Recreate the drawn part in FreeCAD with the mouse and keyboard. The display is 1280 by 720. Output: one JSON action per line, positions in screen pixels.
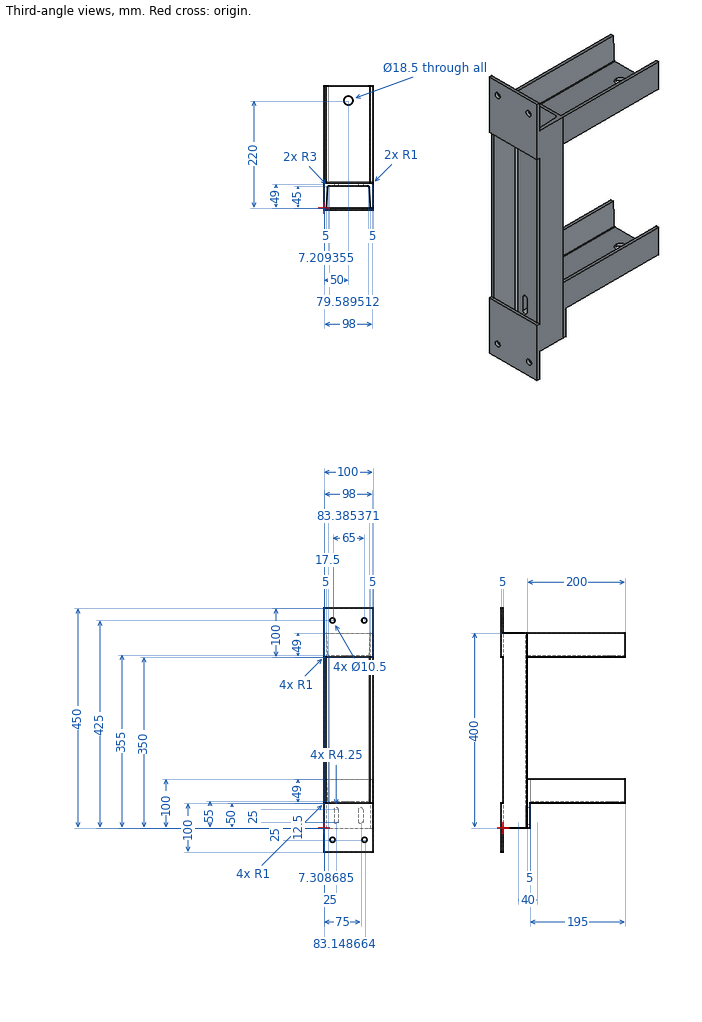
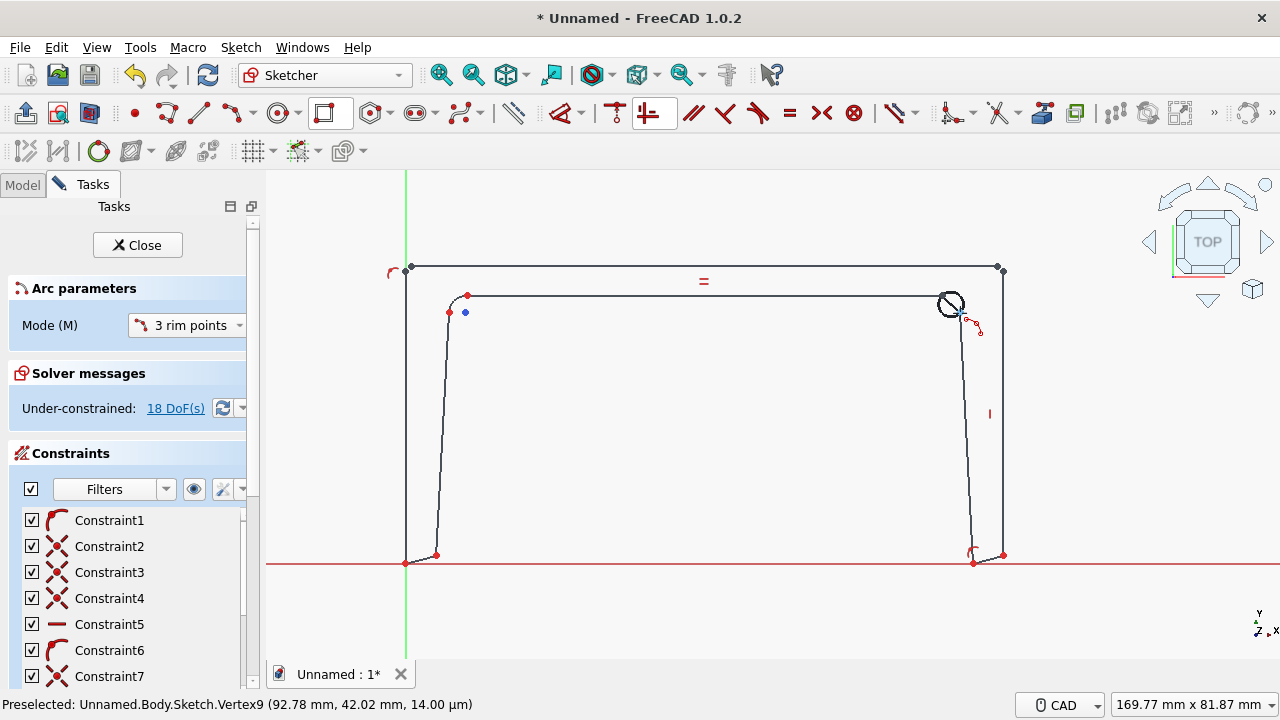
{"action": "scroll", "coordinate": [955, 300], "scroll_direction": "up", "scroll_amount": 6}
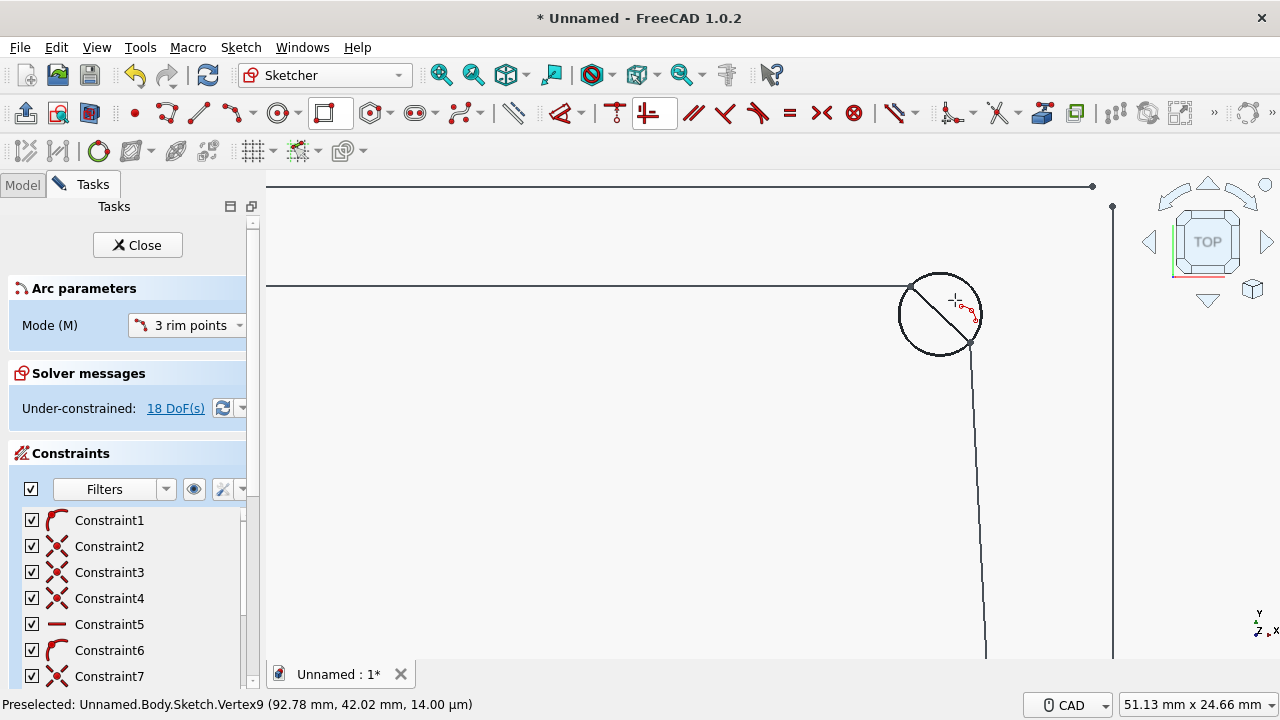
{"action": "left_click", "coordinate": [952, 300]}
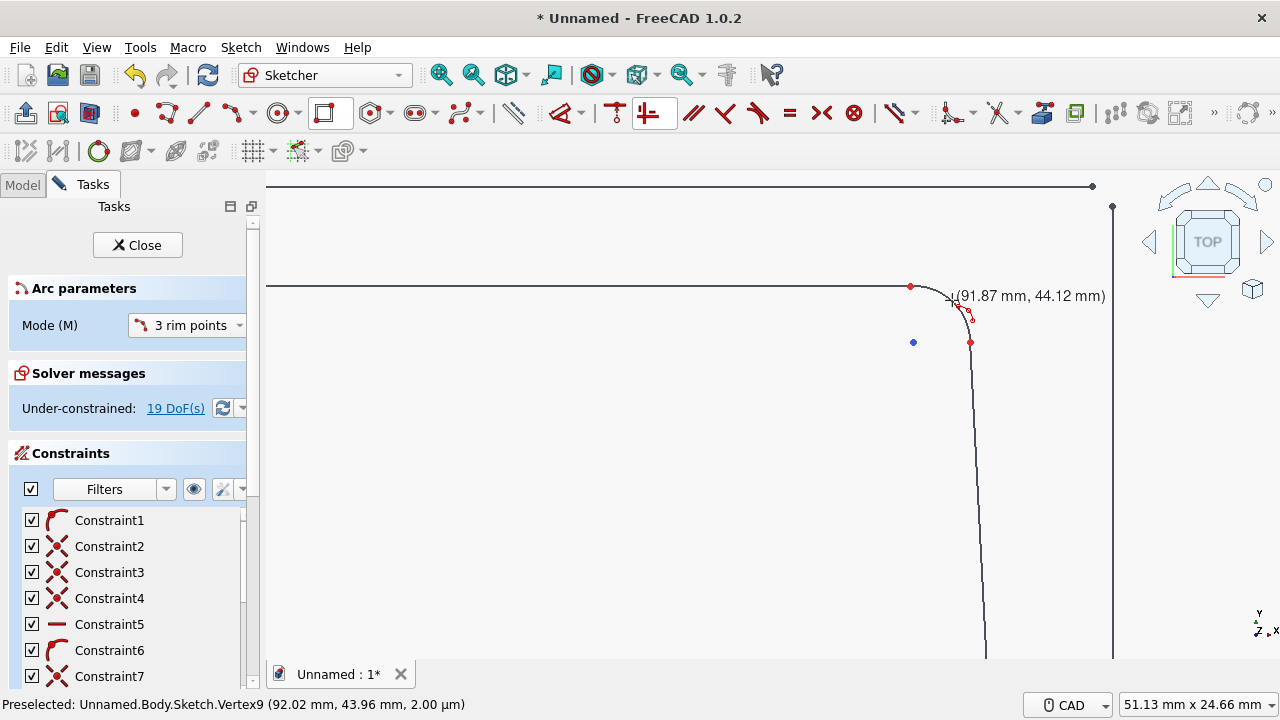
{"action": "left_click", "coordinate": [1113, 206]}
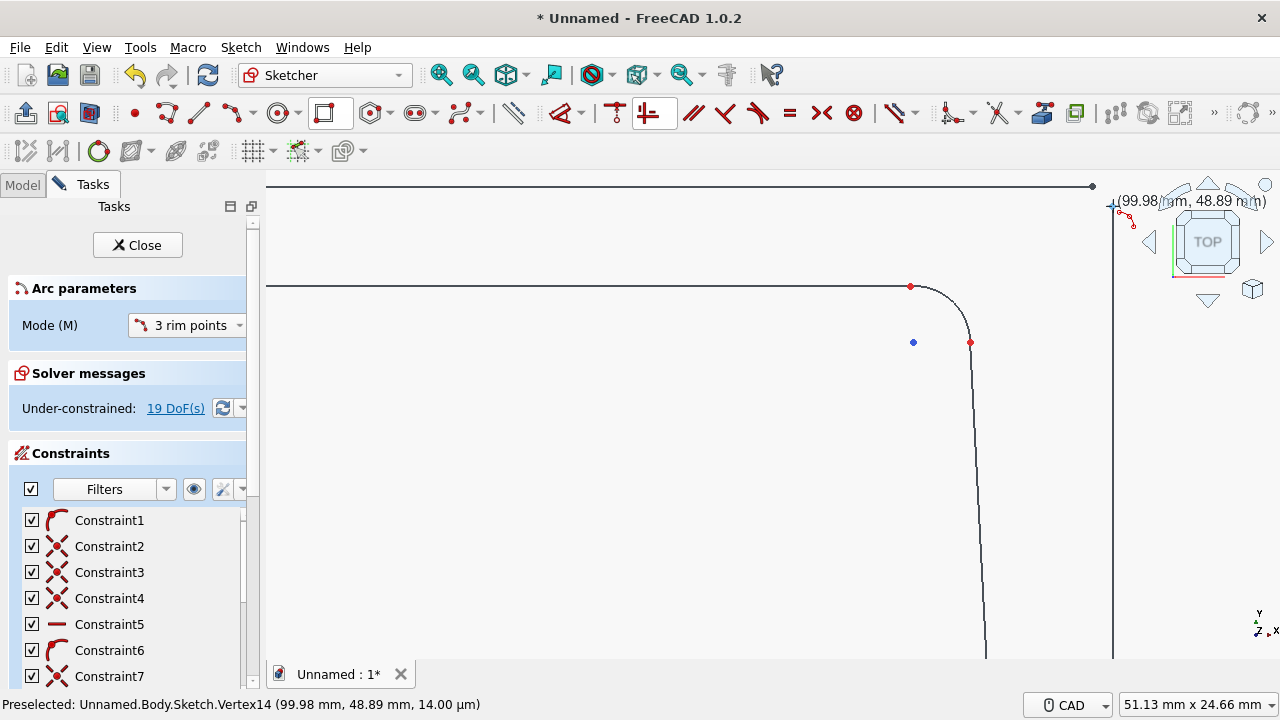
{"action": "scroll", "coordinate": [956, 300], "scroll_direction": "down", "scroll_amount": 6}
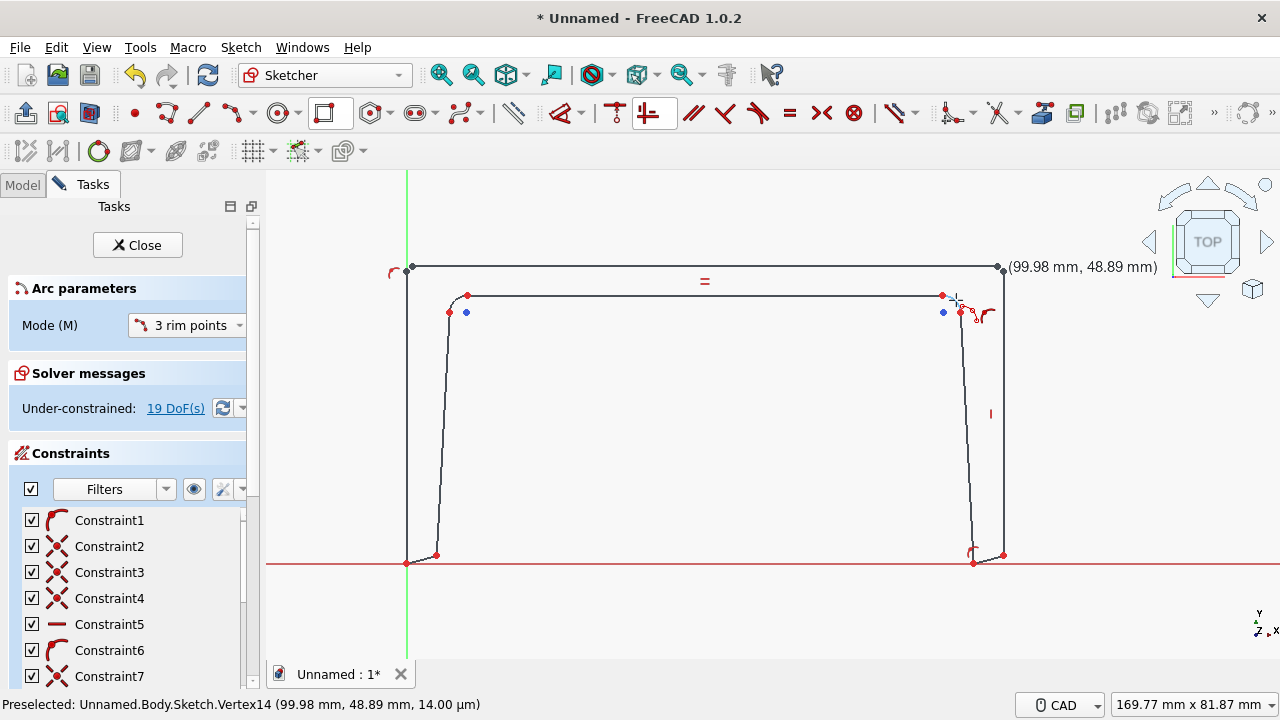
{"action": "scroll", "coordinate": [998, 265], "scroll_direction": "up", "scroll_amount": 4}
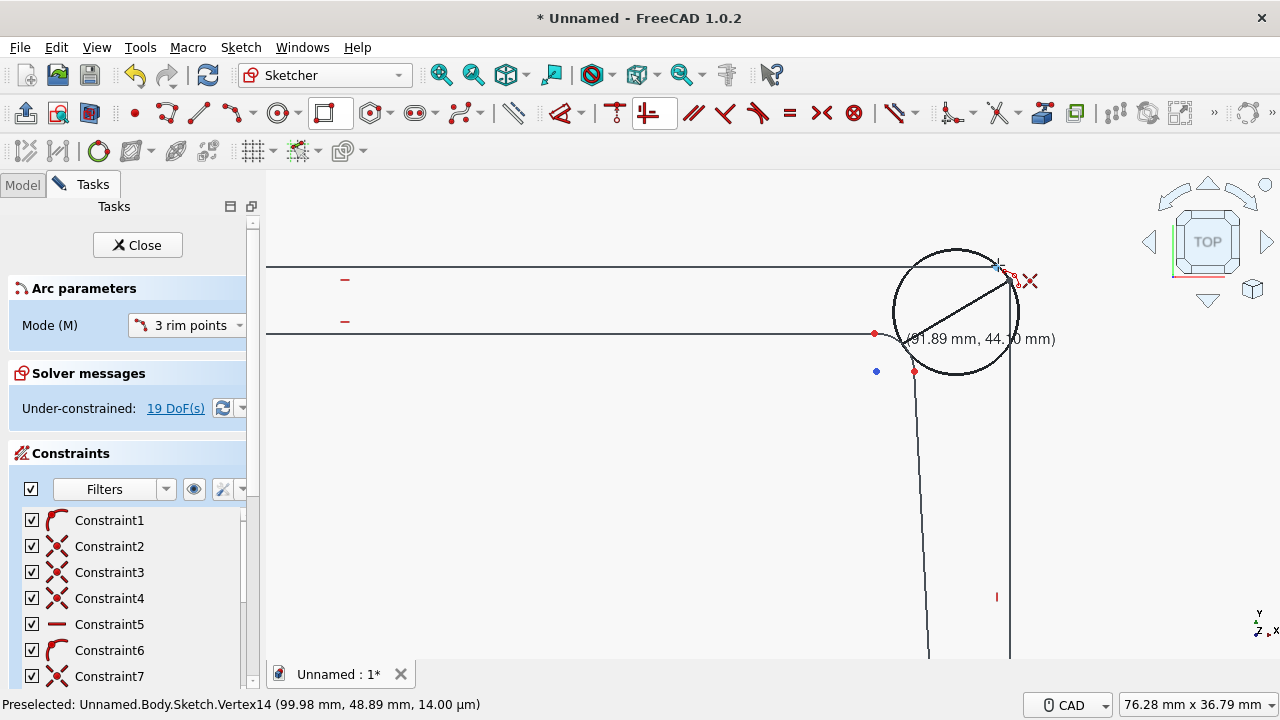
{"action": "left_click", "coordinate": [996, 267]}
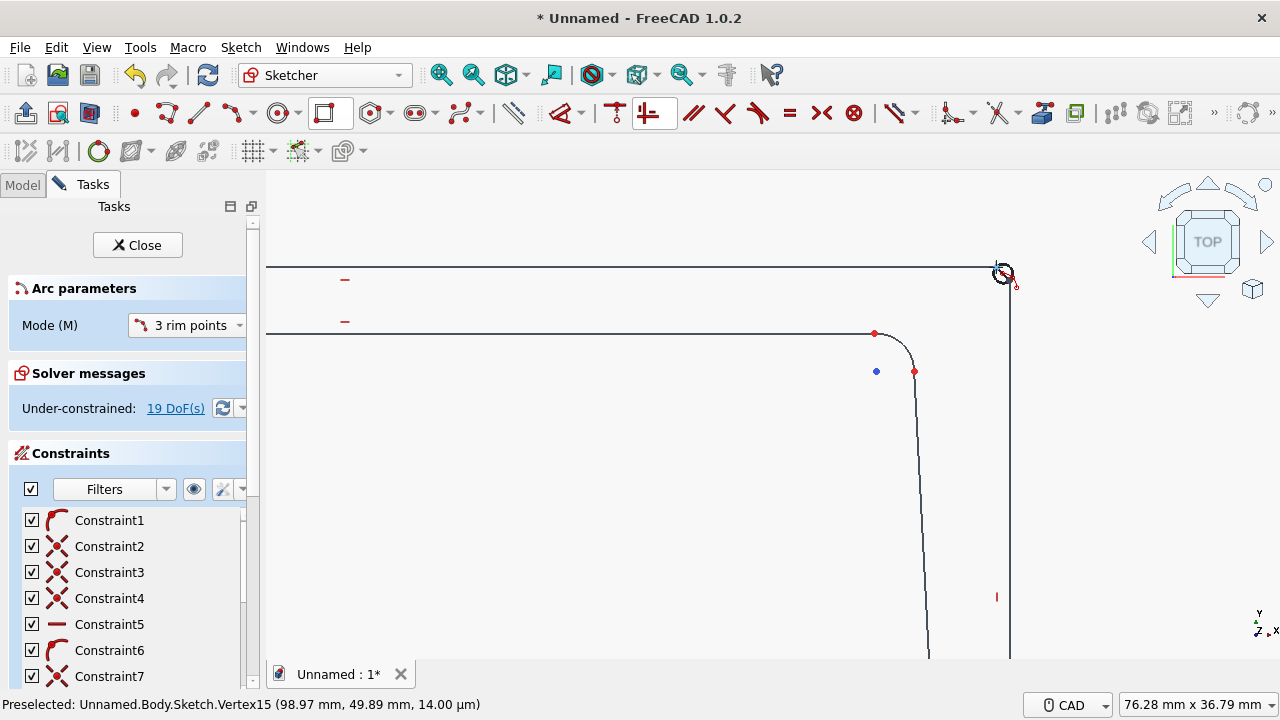
{"action": "scroll", "coordinate": [1006, 269], "scroll_direction": "up", "scroll_amount": 8}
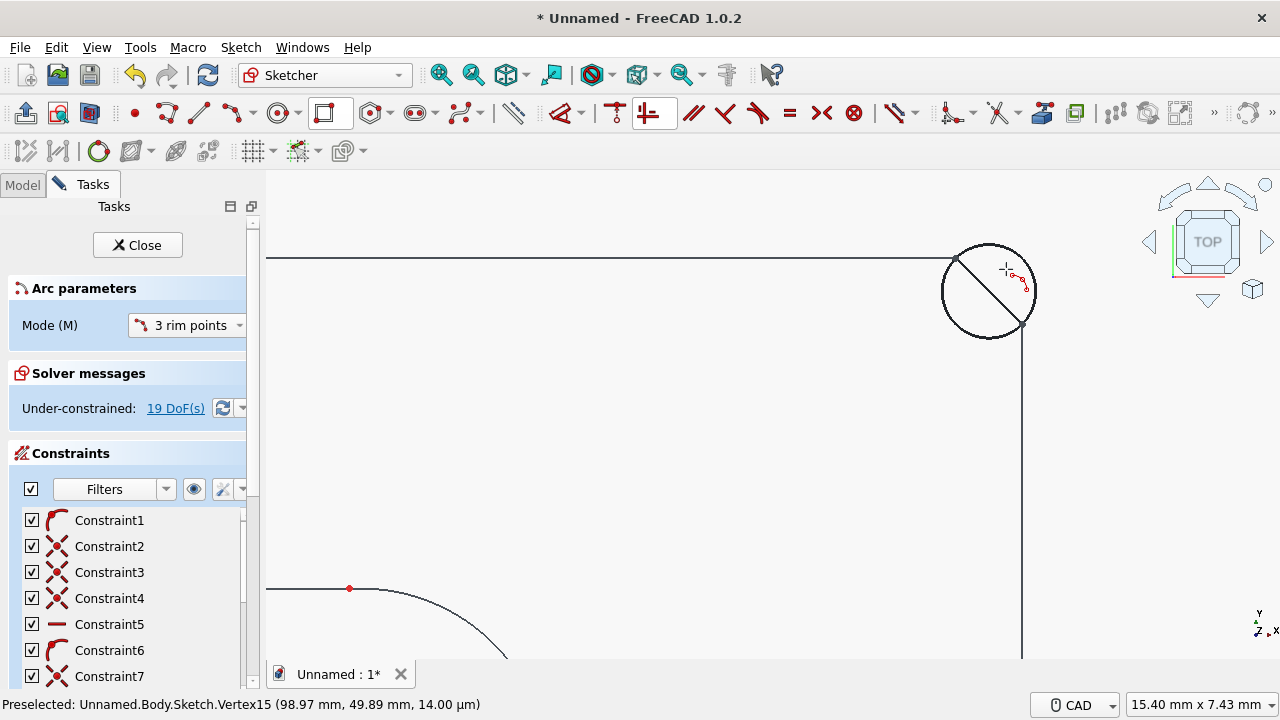
{"action": "left_click", "coordinate": [1004, 270]}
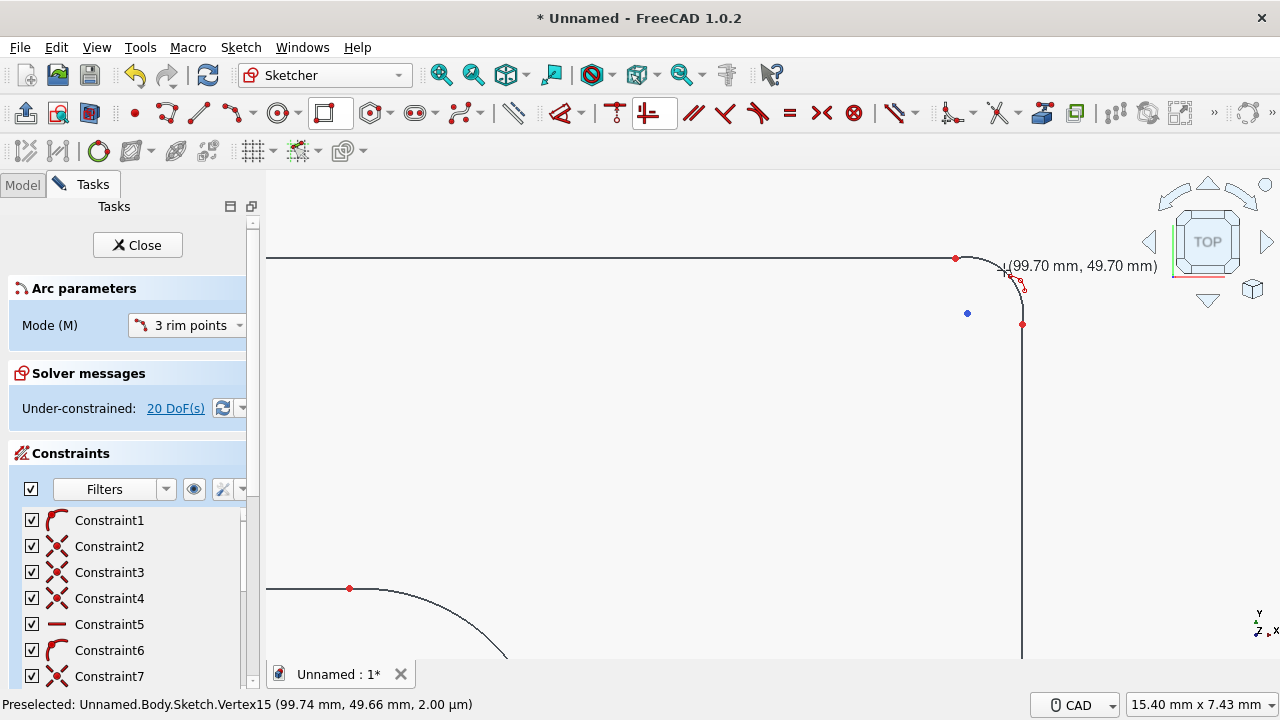
{"action": "scroll", "coordinate": [1001, 267], "scroll_direction": "down", "scroll_amount": 12}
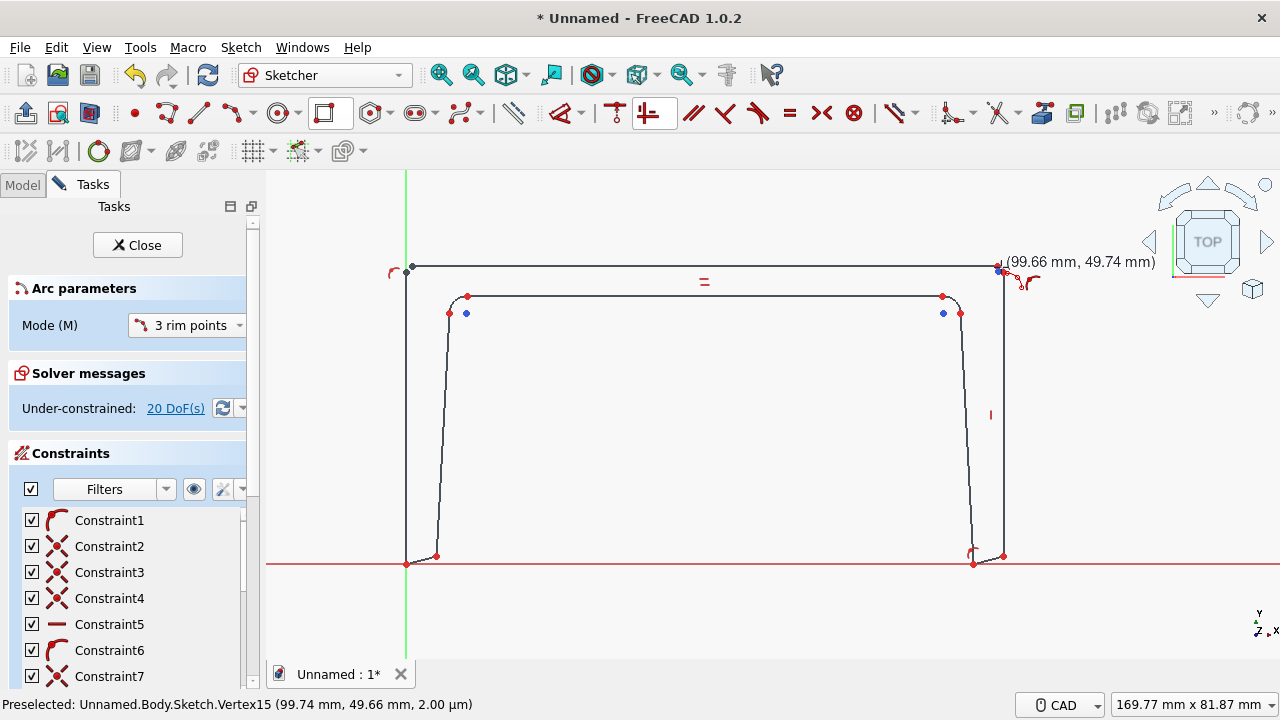
{"action": "scroll", "coordinate": [412, 266], "scroll_direction": "up", "scroll_amount": 5}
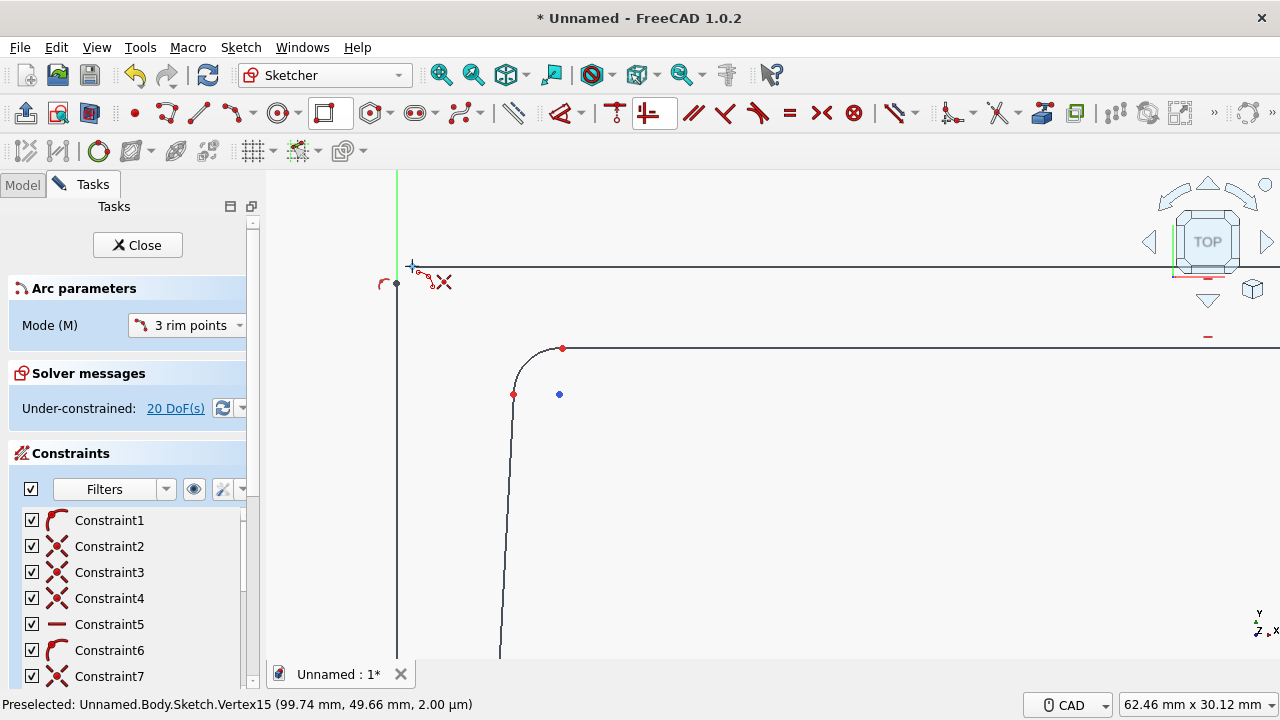
{"action": "left_click", "coordinate": [413, 267]}
{"action": "left_click", "coordinate": [397, 283]}